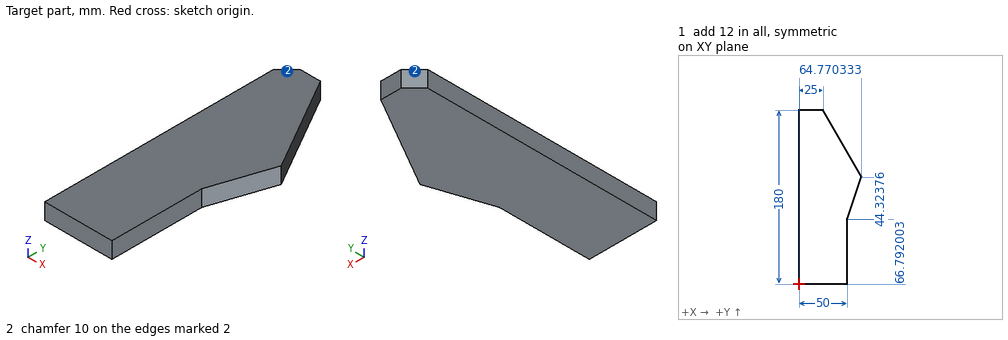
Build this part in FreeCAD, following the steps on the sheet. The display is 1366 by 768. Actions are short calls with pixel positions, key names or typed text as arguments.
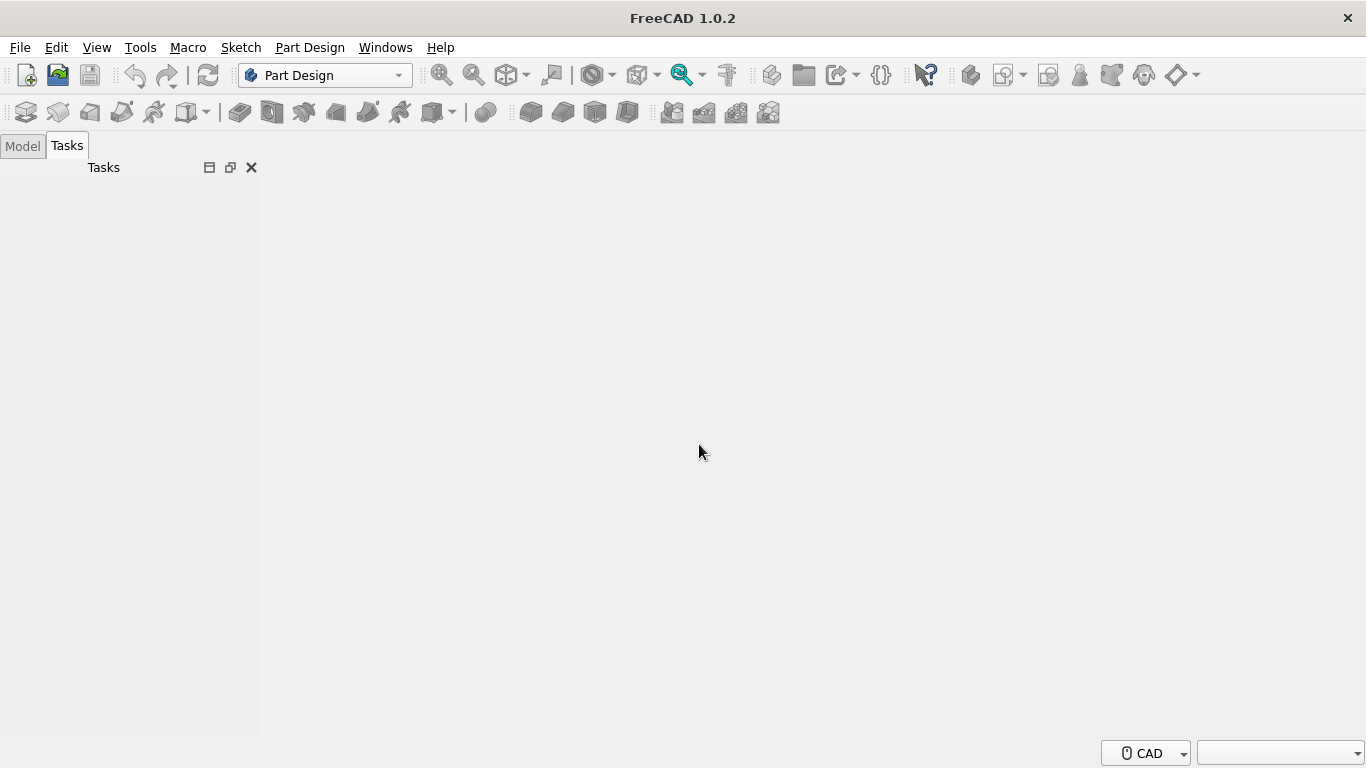
key(ctrl+n)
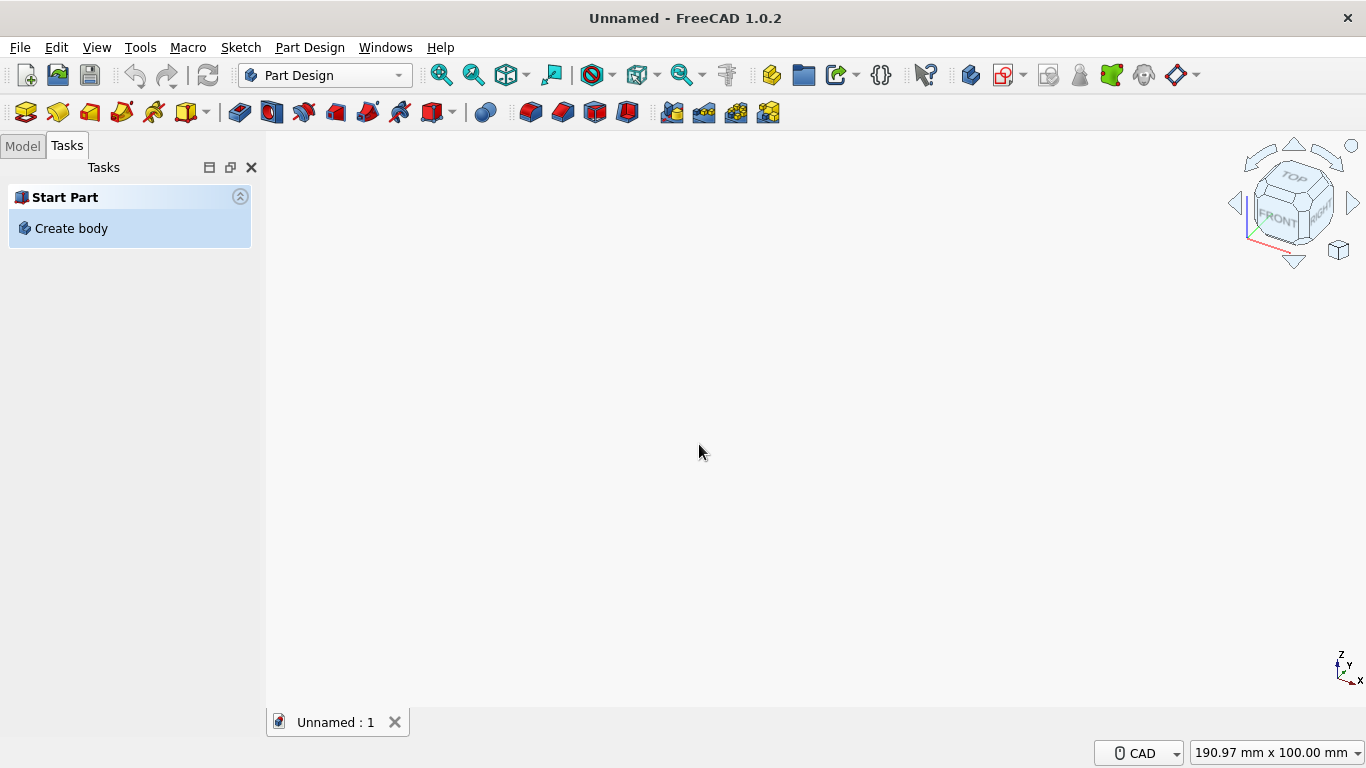
click(1004, 76)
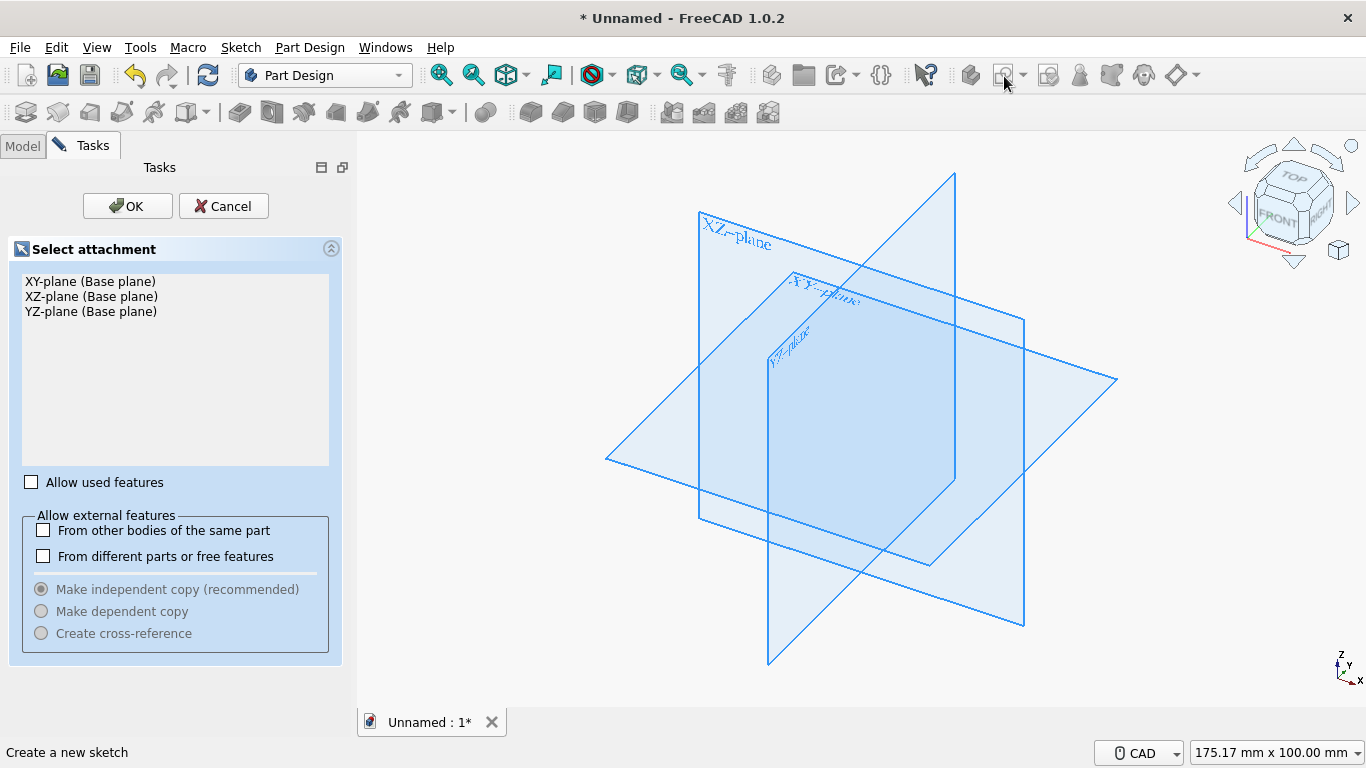
click(82, 282)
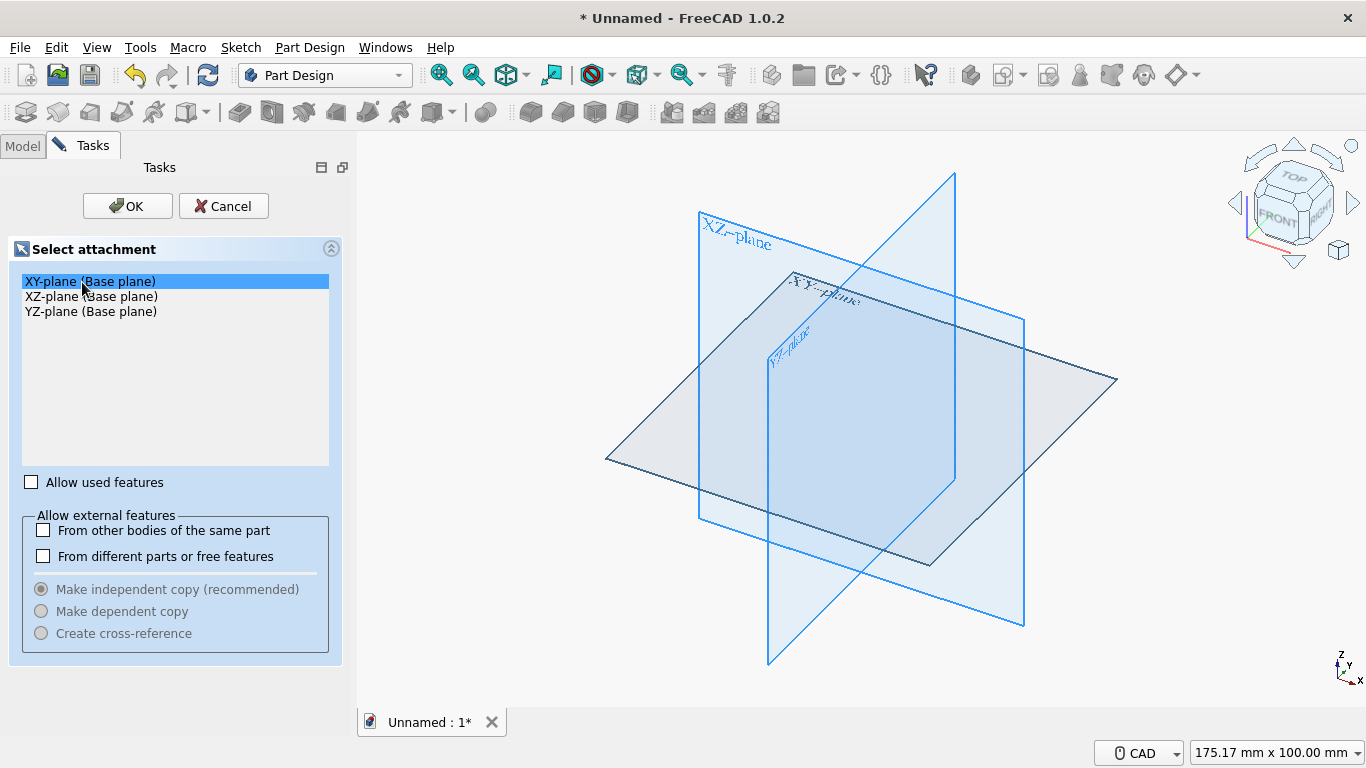
click(128, 206)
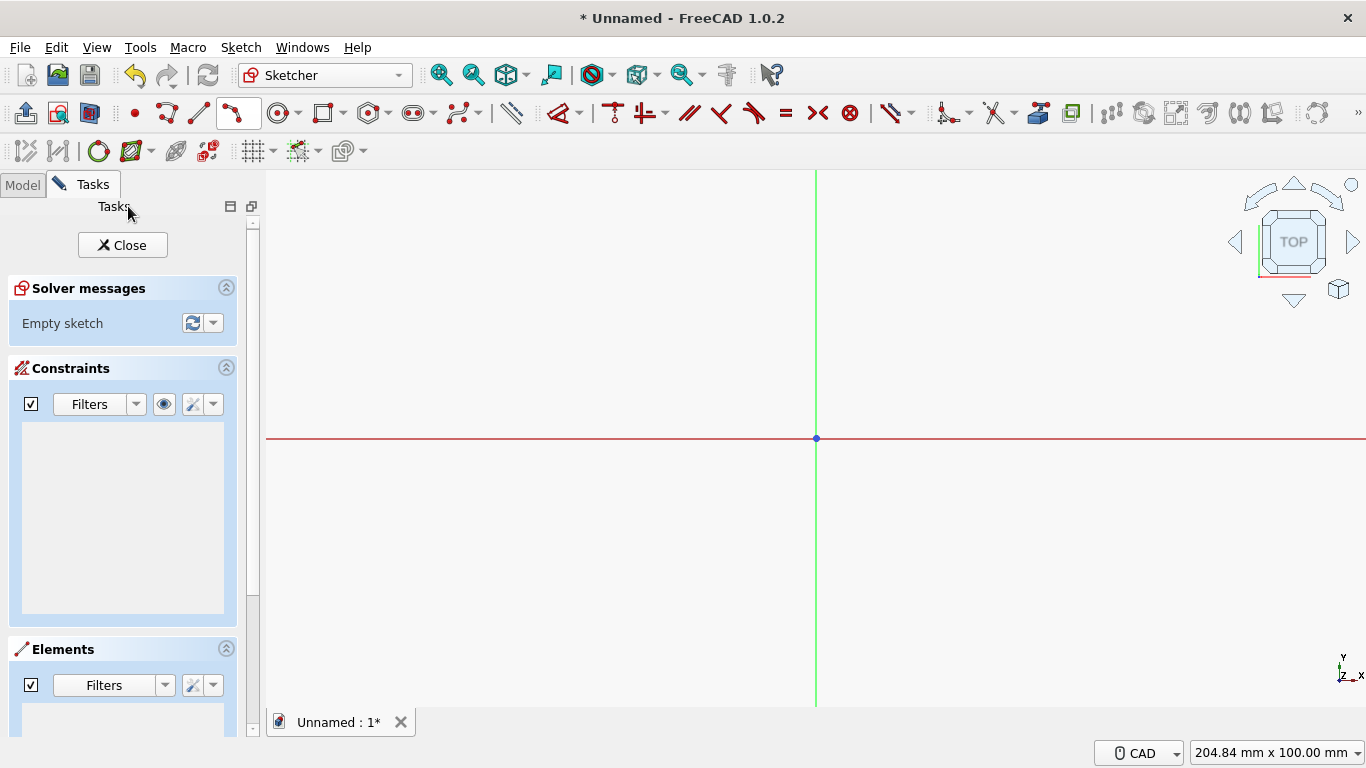
scroll(606, 679, down, 5)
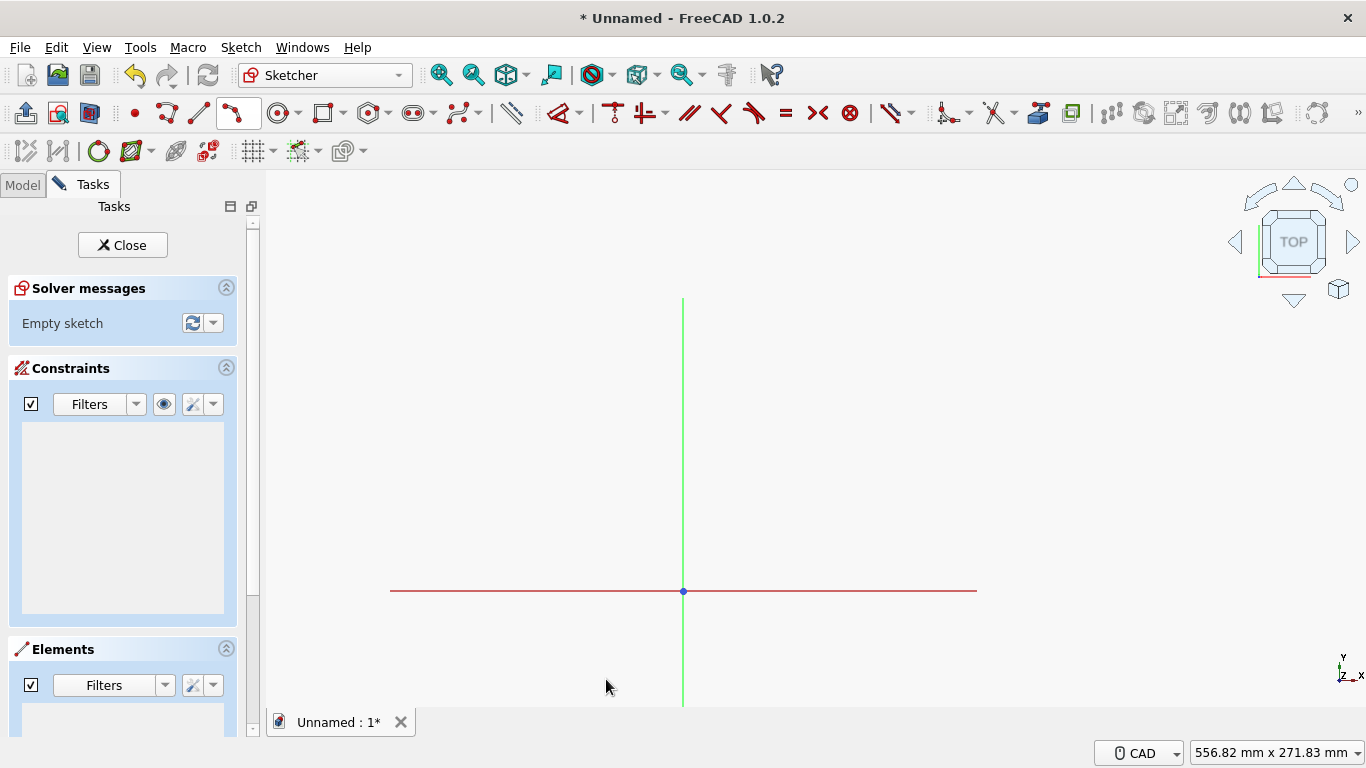
click(168, 114)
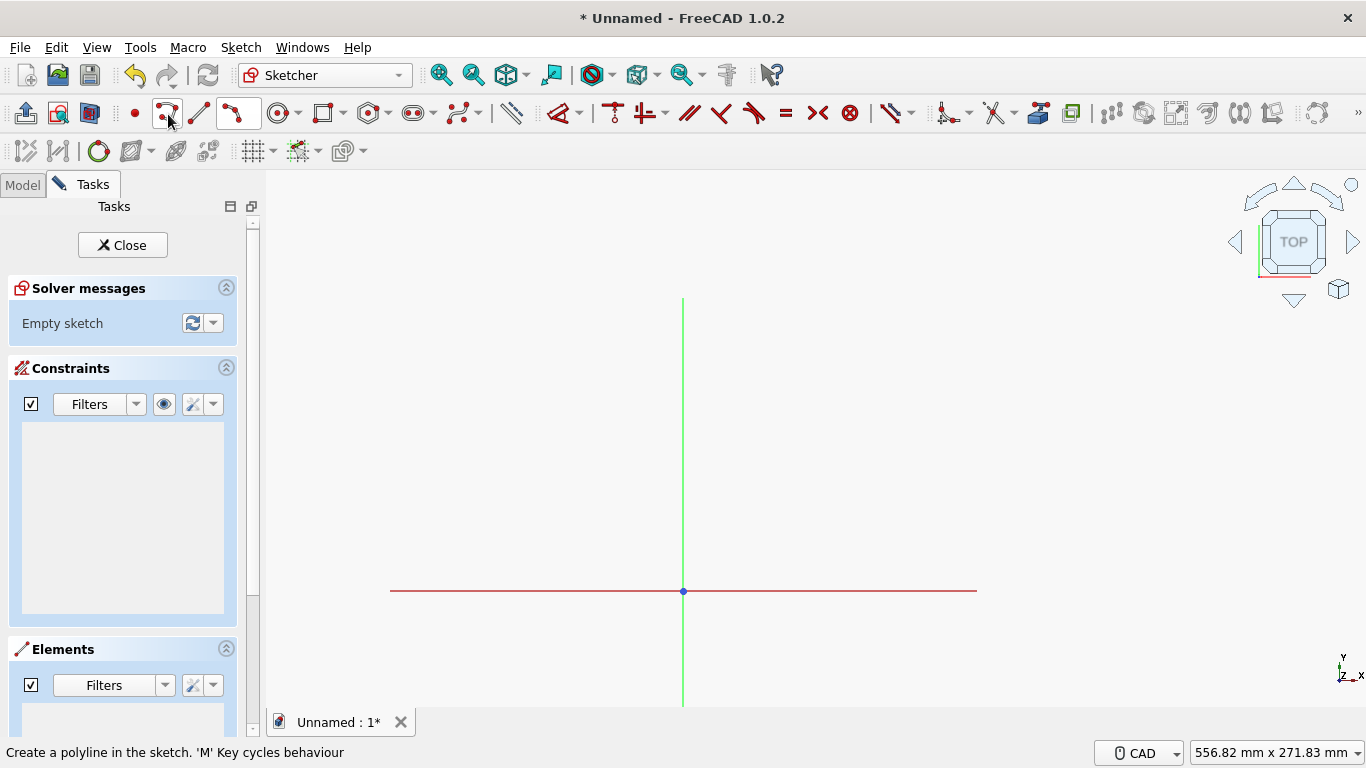
click(683, 591)
click(782, 582)
click(782, 459)
click(811, 372)
click(733, 236)
click(692, 236)
click(683, 591)
key(Escape)
key(Escape)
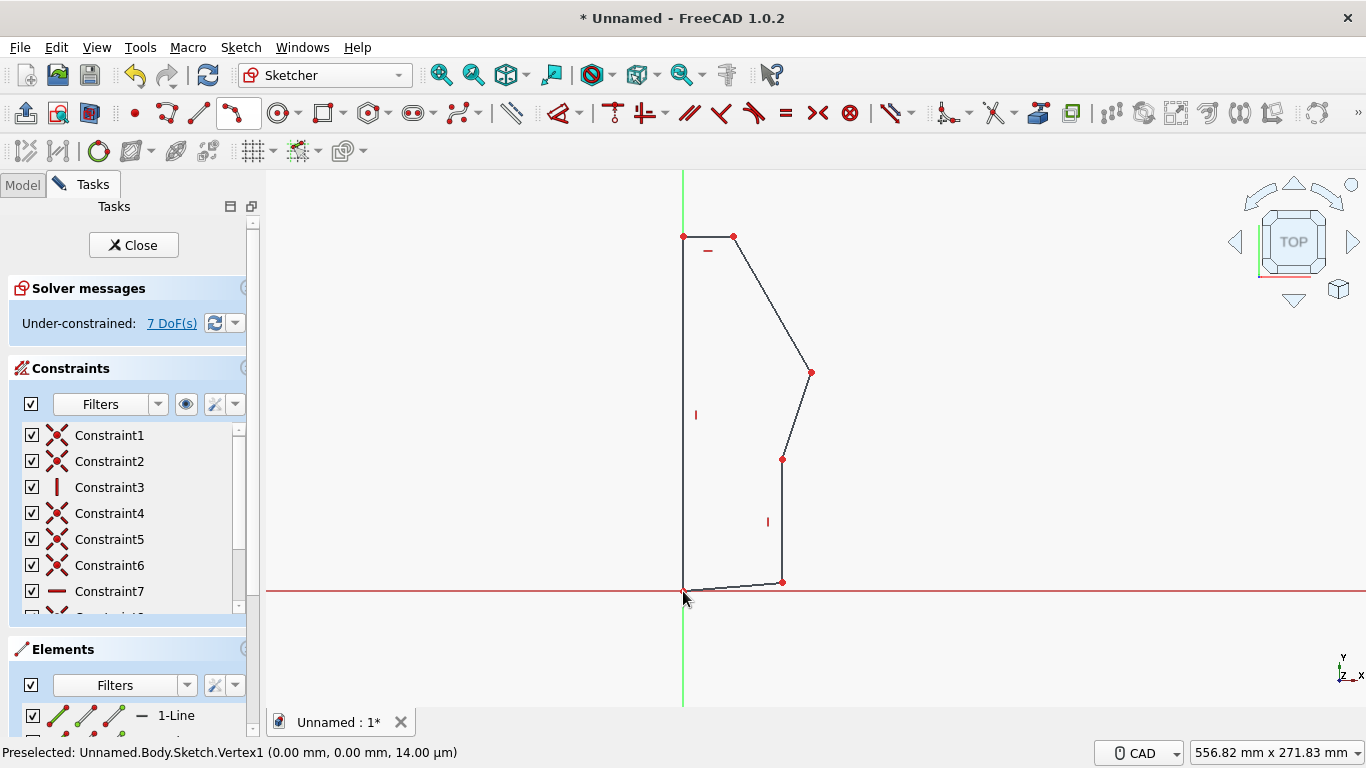
click(713, 589)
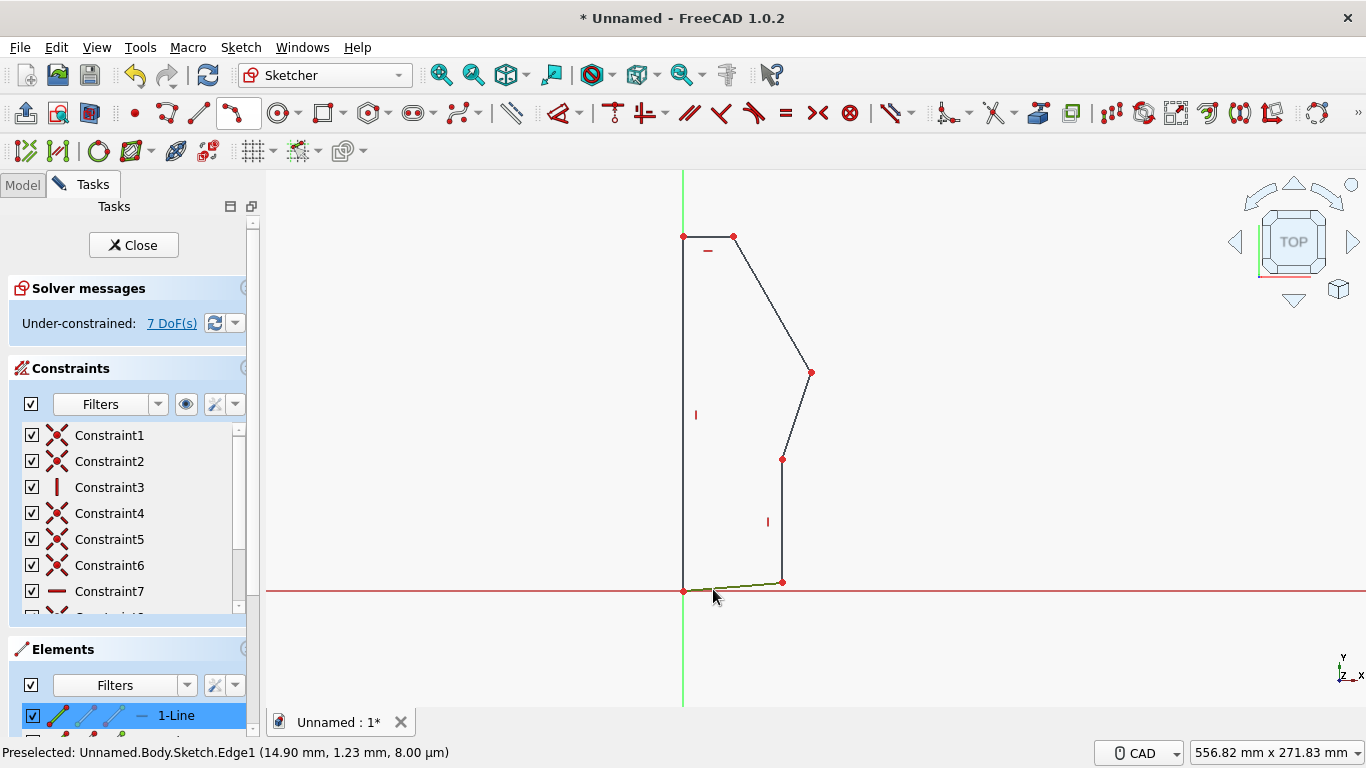
key(h)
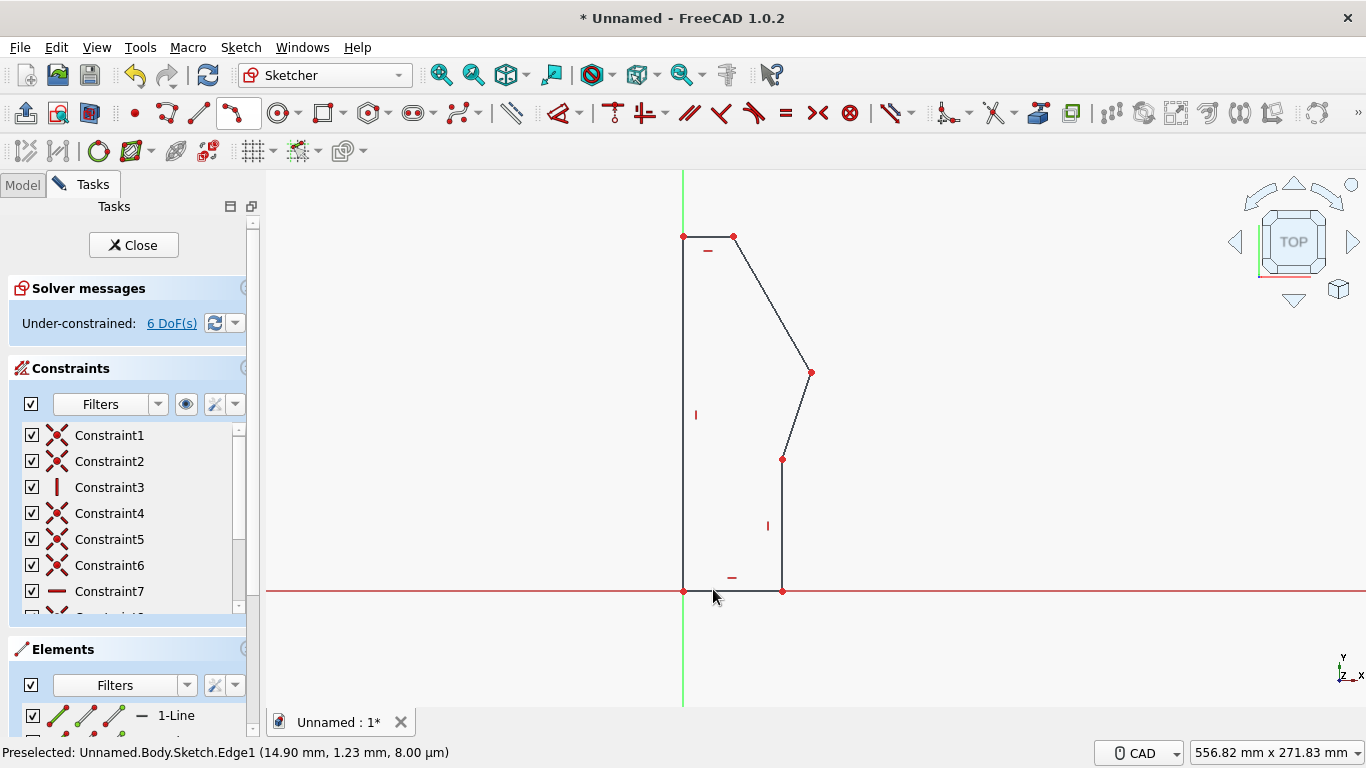
click(558, 114)